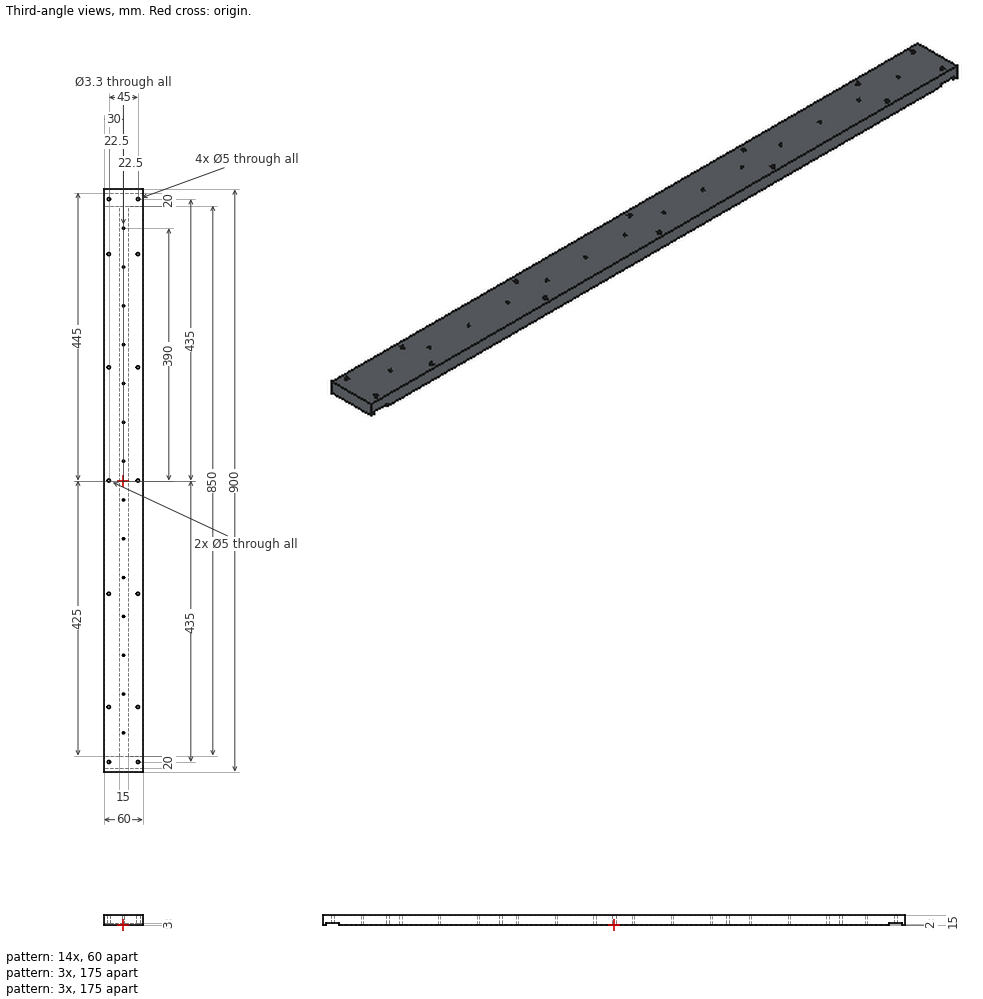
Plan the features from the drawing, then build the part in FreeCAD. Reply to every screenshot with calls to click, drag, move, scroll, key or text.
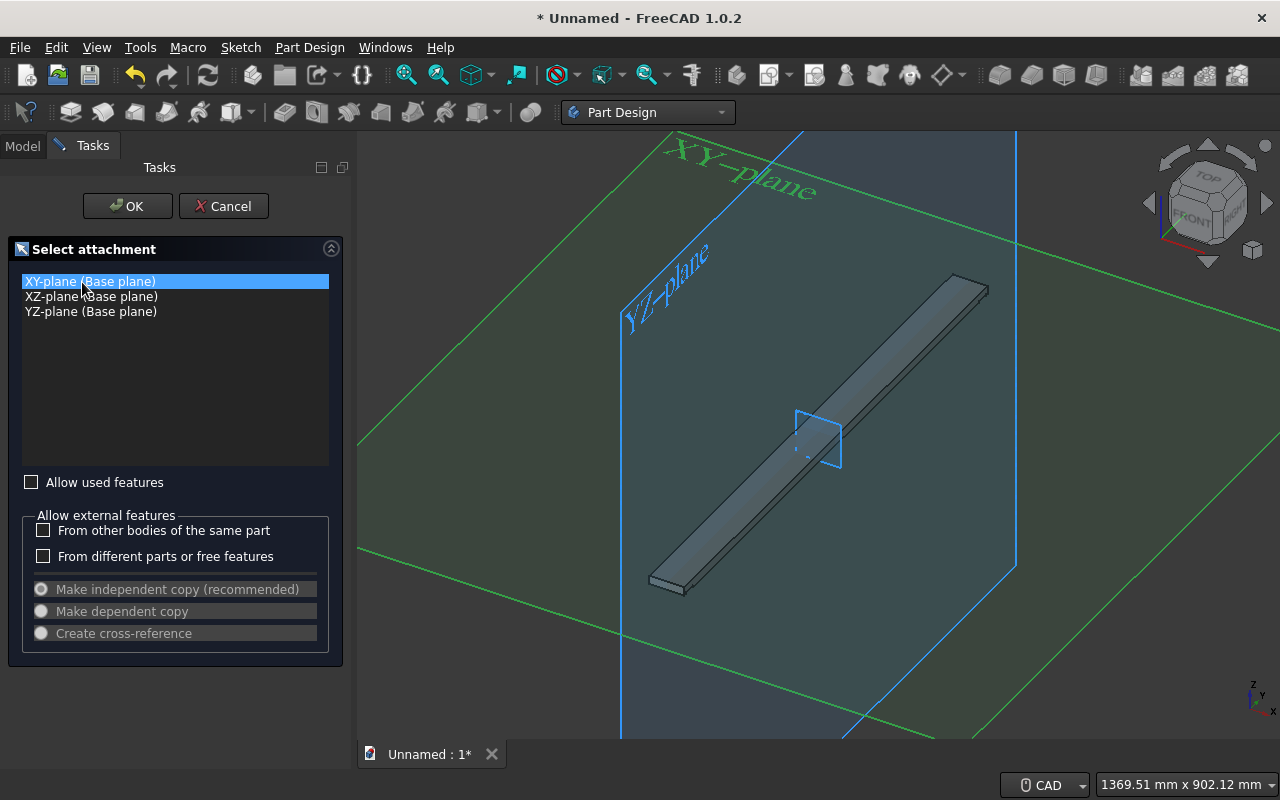
click(128, 206)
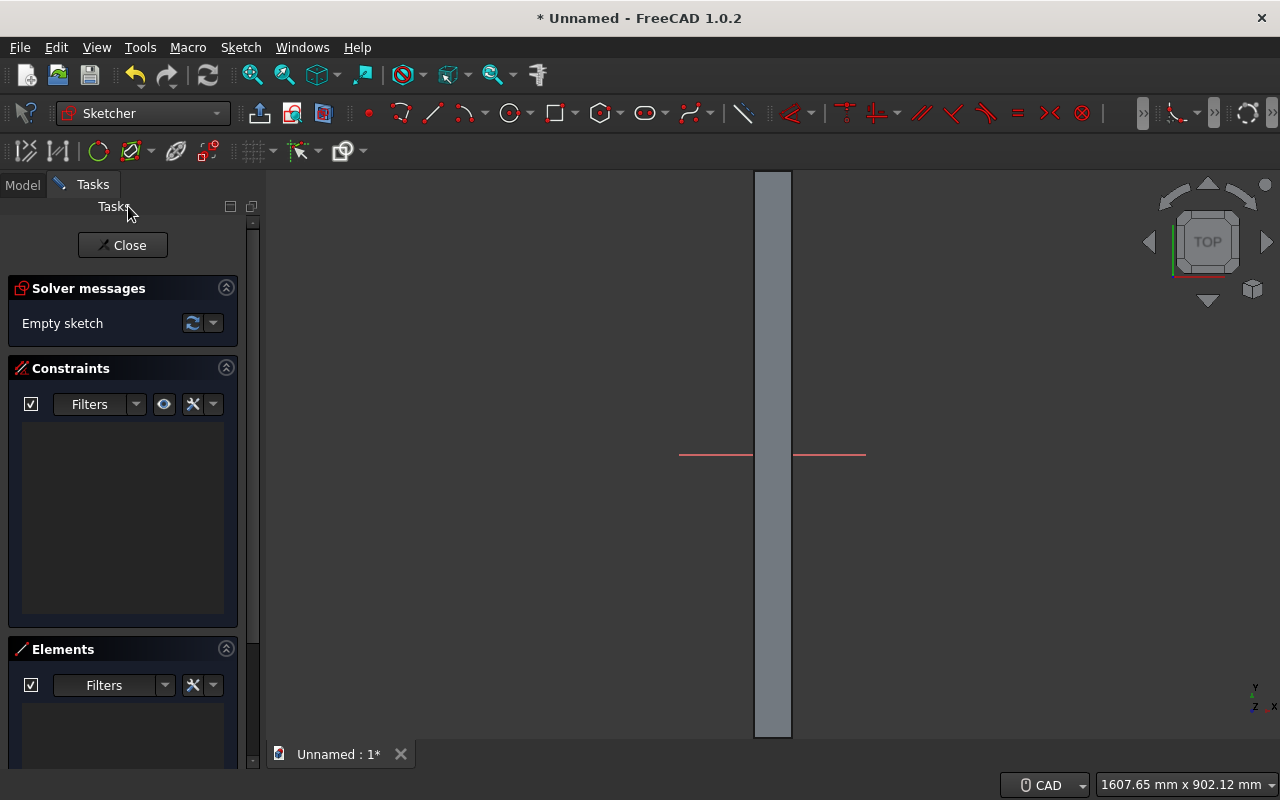
key(q)
key(s)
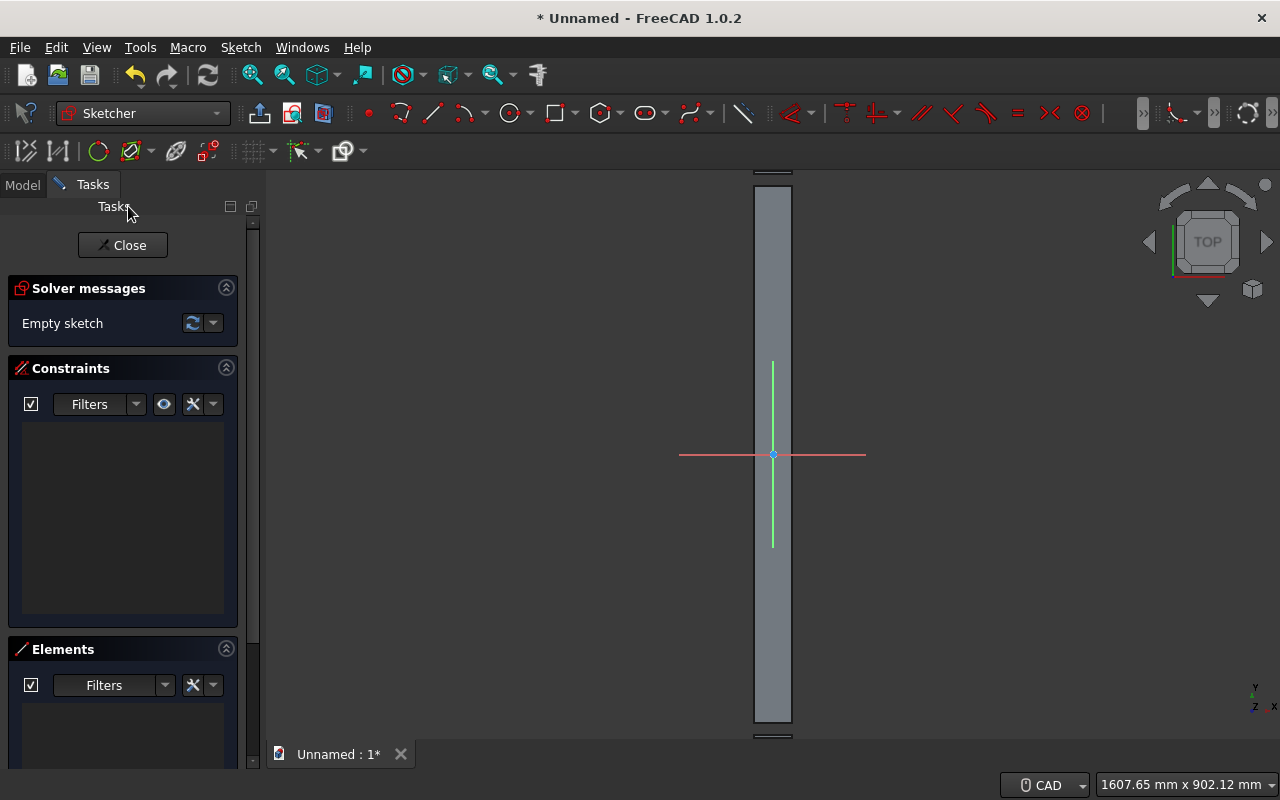
scroll(565, 455, down, 2)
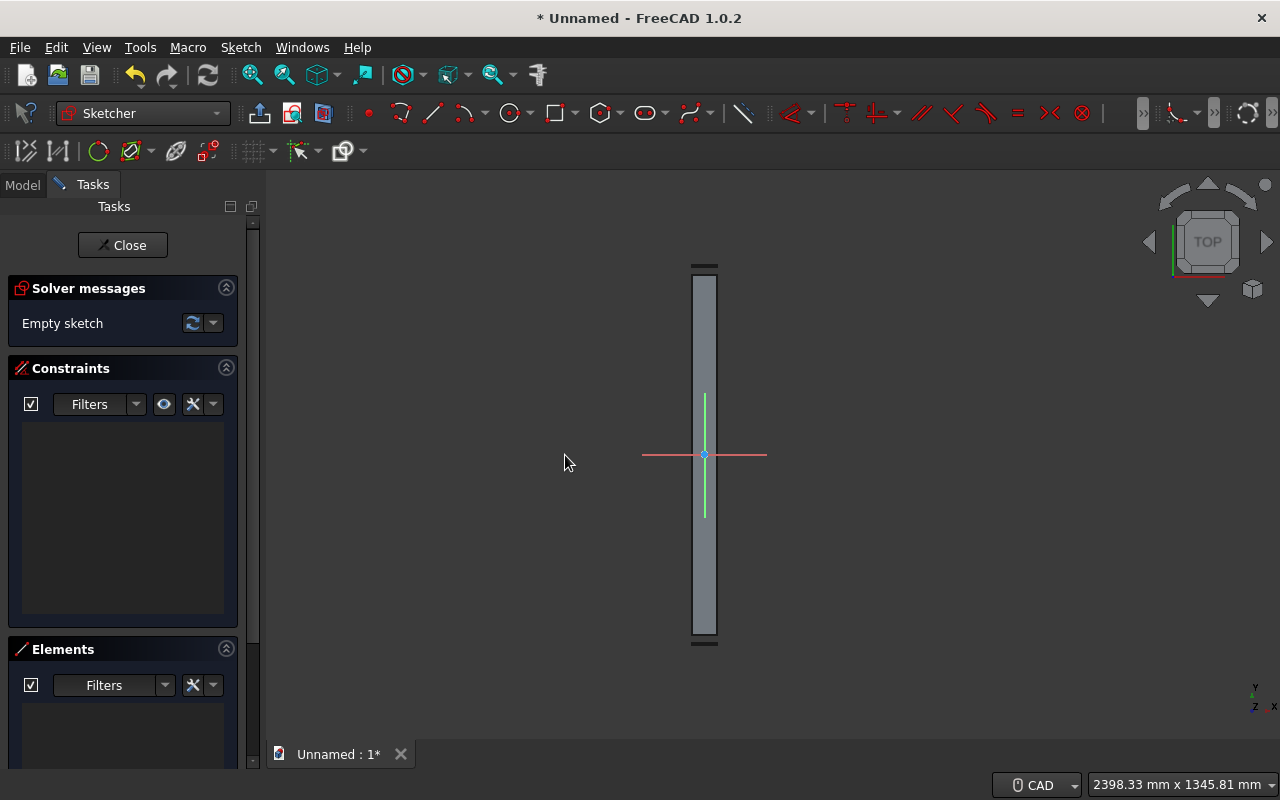
key(g)
key(v)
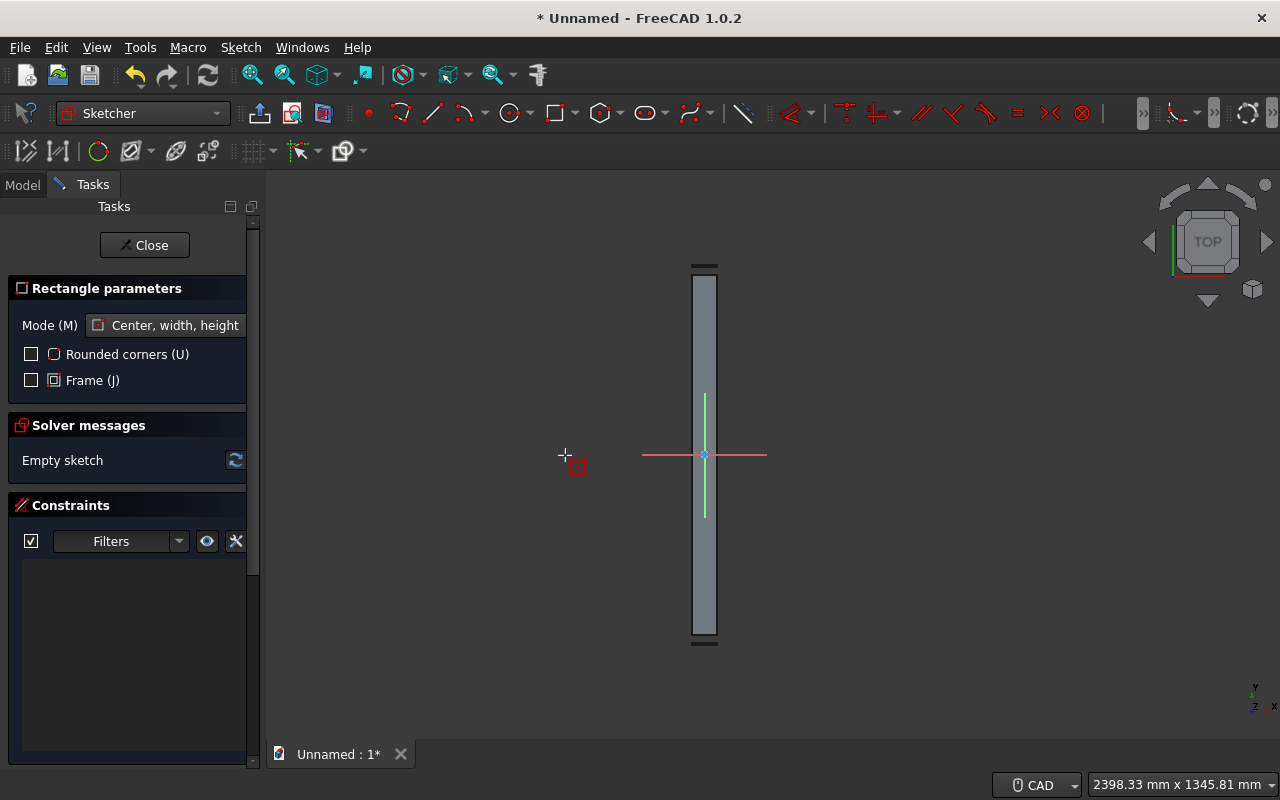
scroll(705, 455, up, 9)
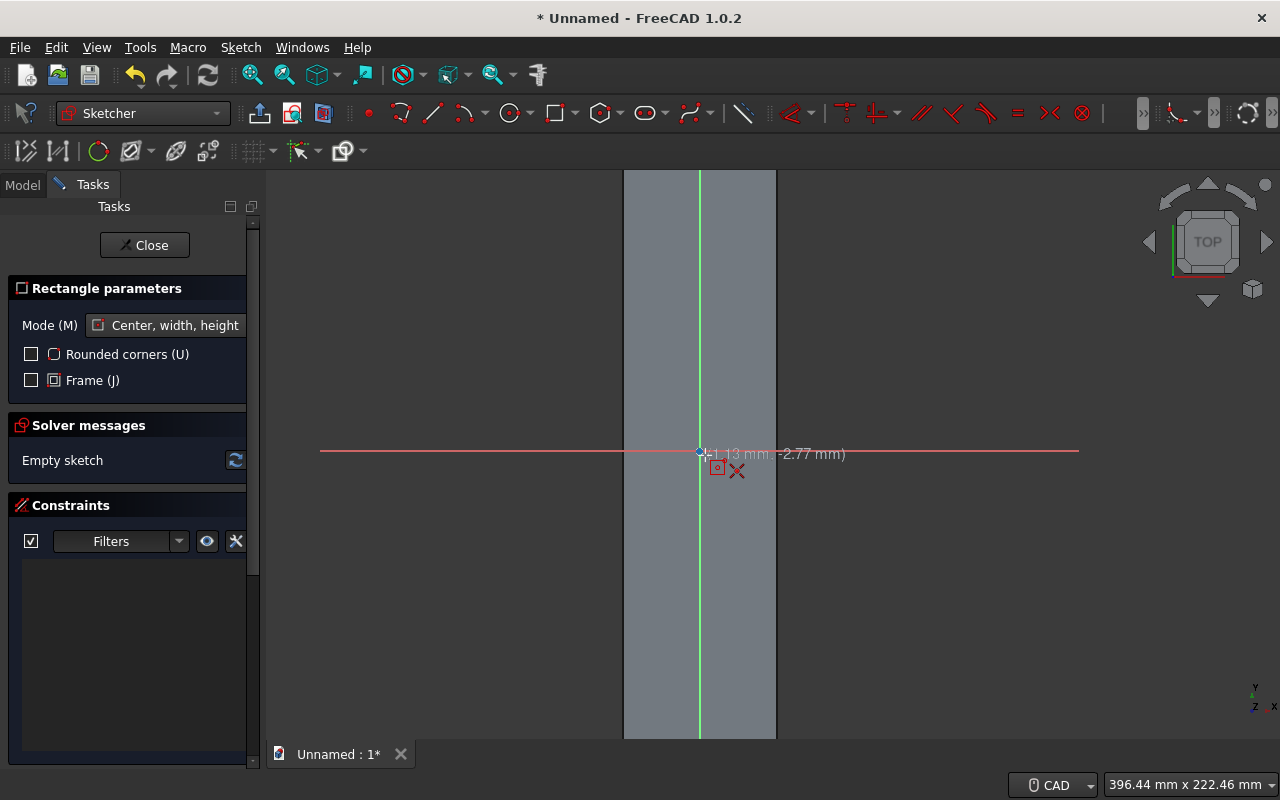
scroll(705, 455, down, 9)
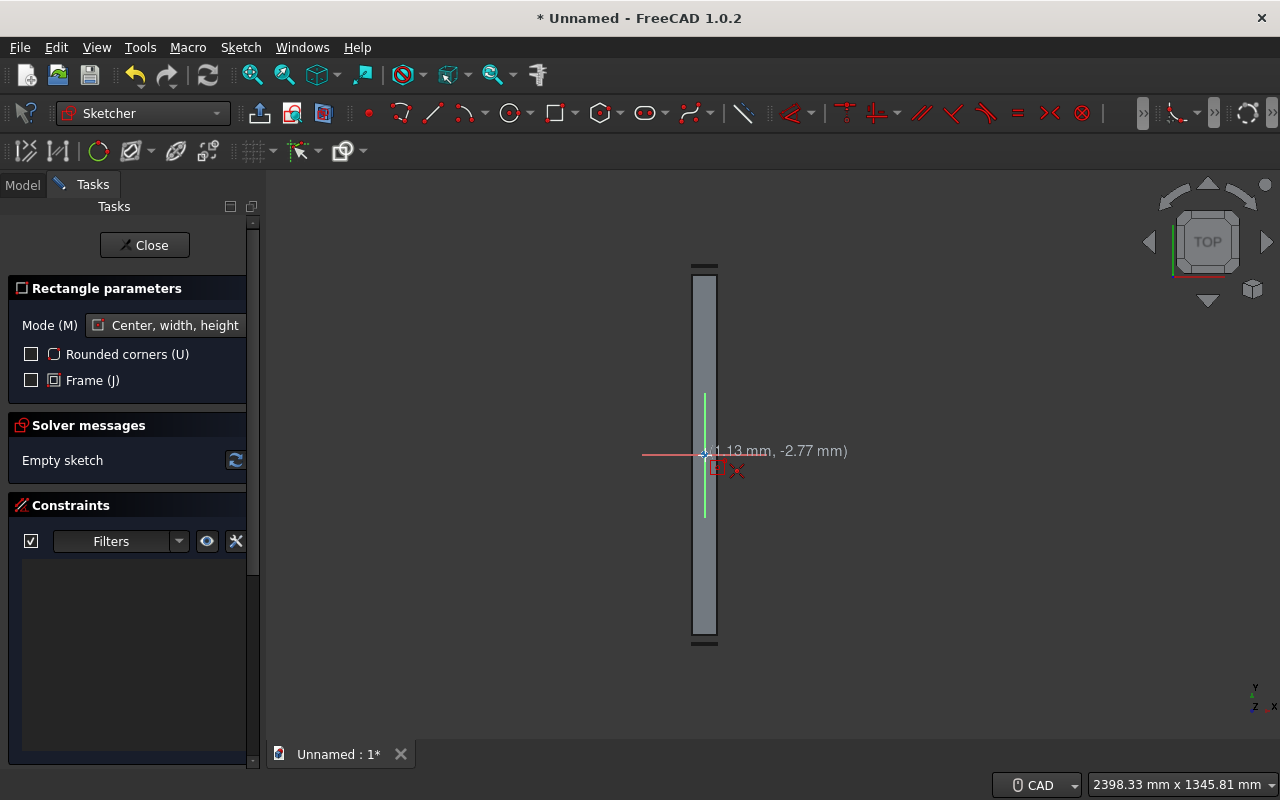
click(705, 455)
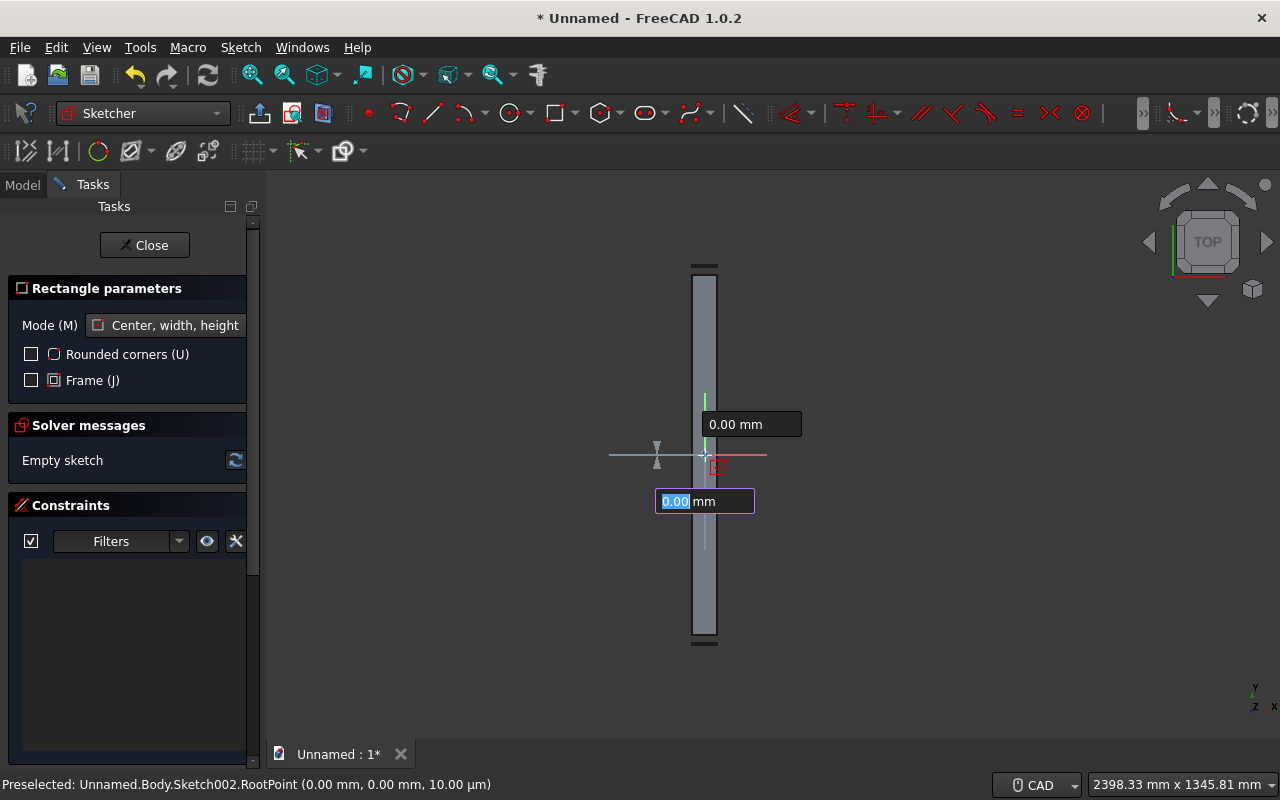
scroll(708, 275, up, 9)
move(704, 275)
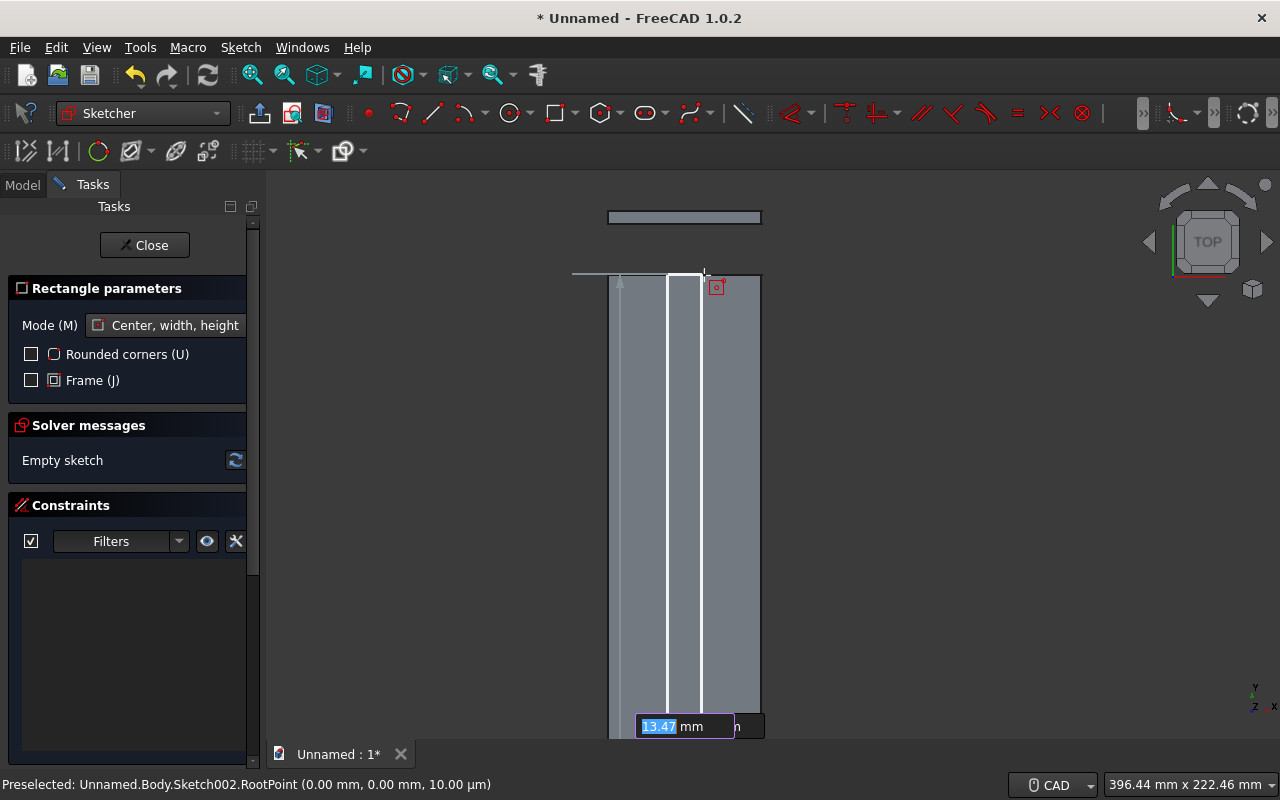
text(15)
key(Tab)
text(850)
key(Return)
key(Escape)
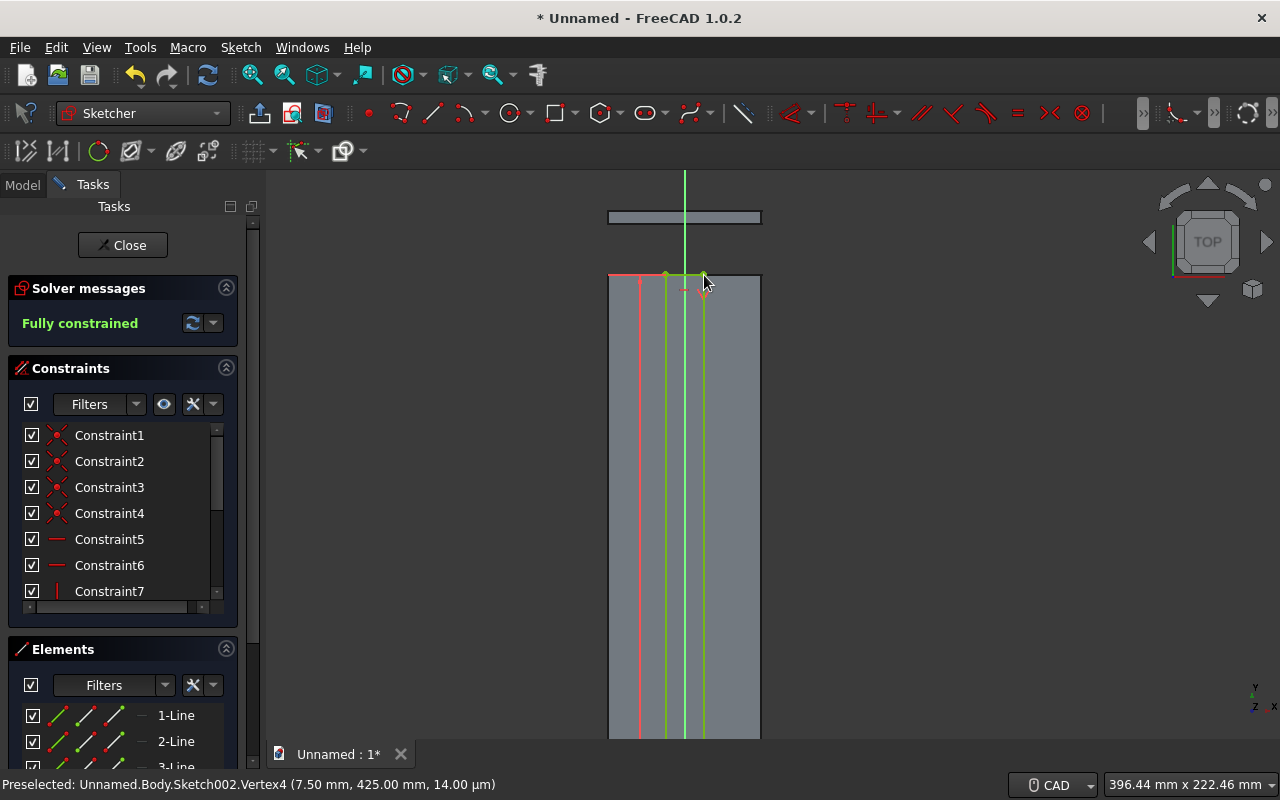
click(123, 245)